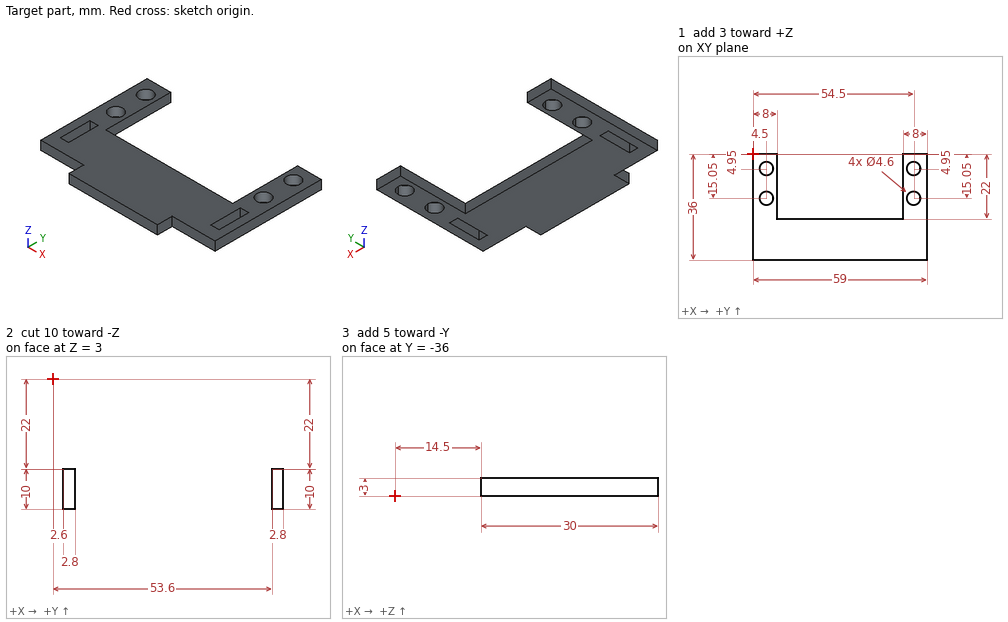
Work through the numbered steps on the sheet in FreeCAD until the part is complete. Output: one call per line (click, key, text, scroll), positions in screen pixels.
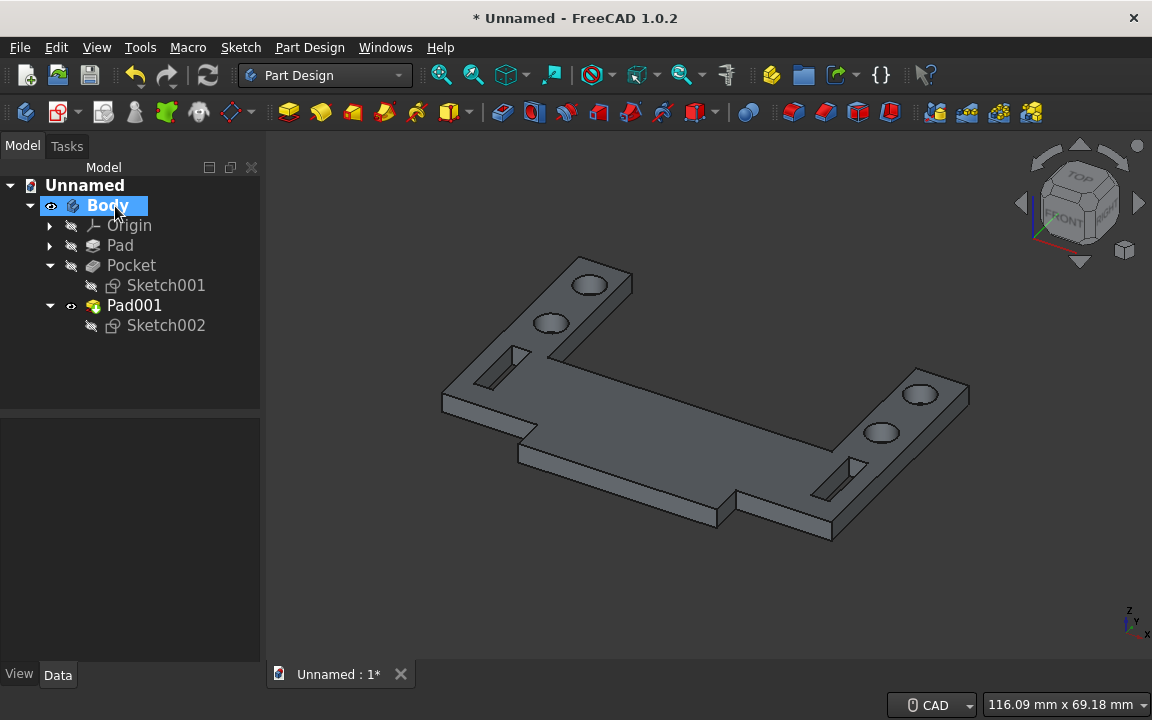
key(0)